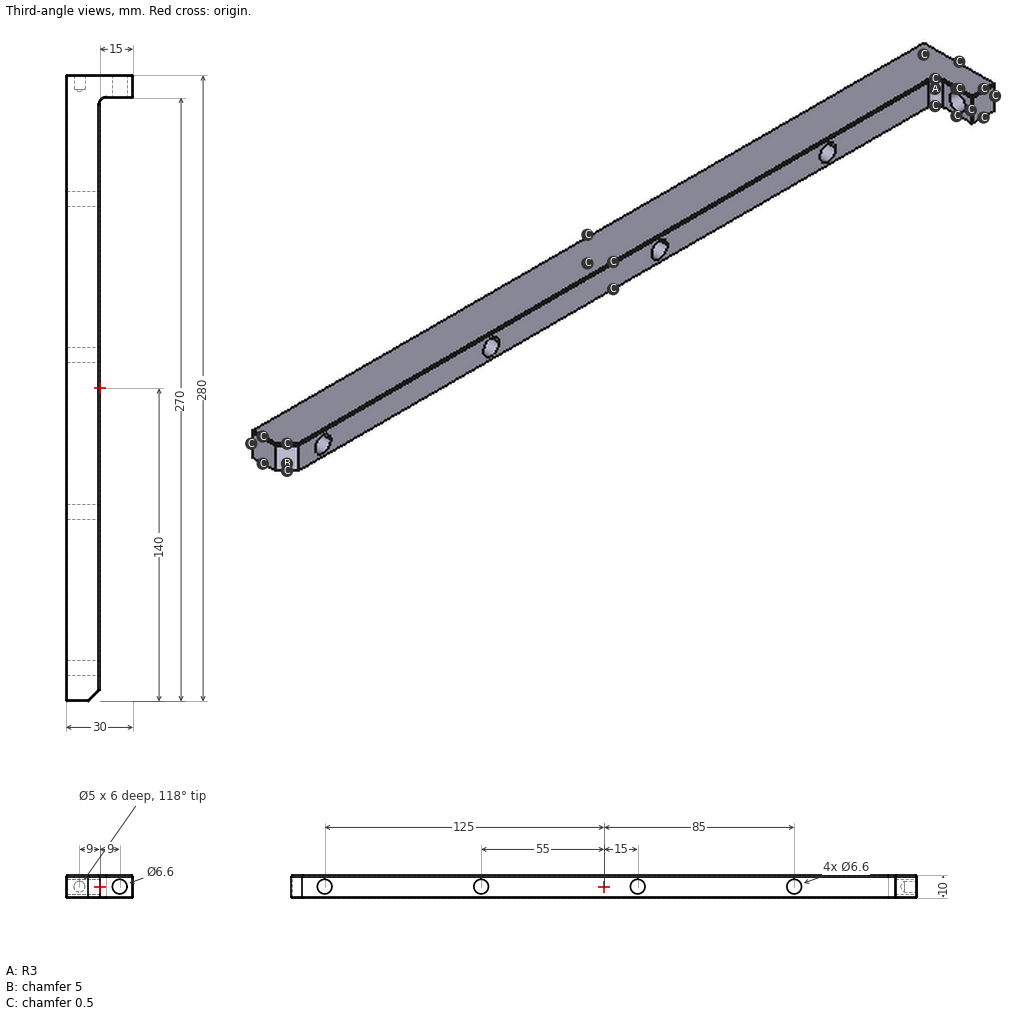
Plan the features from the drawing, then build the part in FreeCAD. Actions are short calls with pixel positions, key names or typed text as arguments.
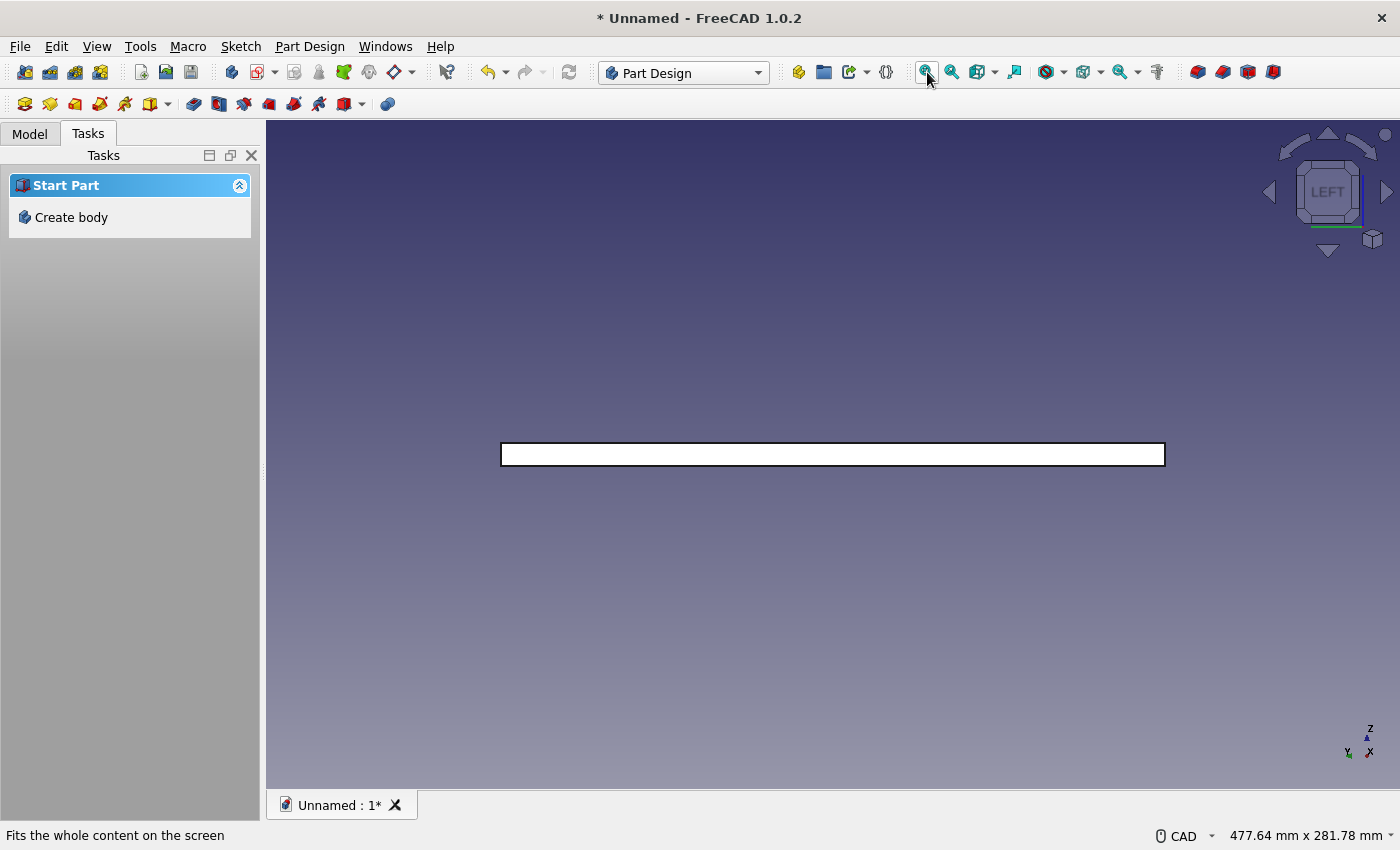
key(v)
key(3)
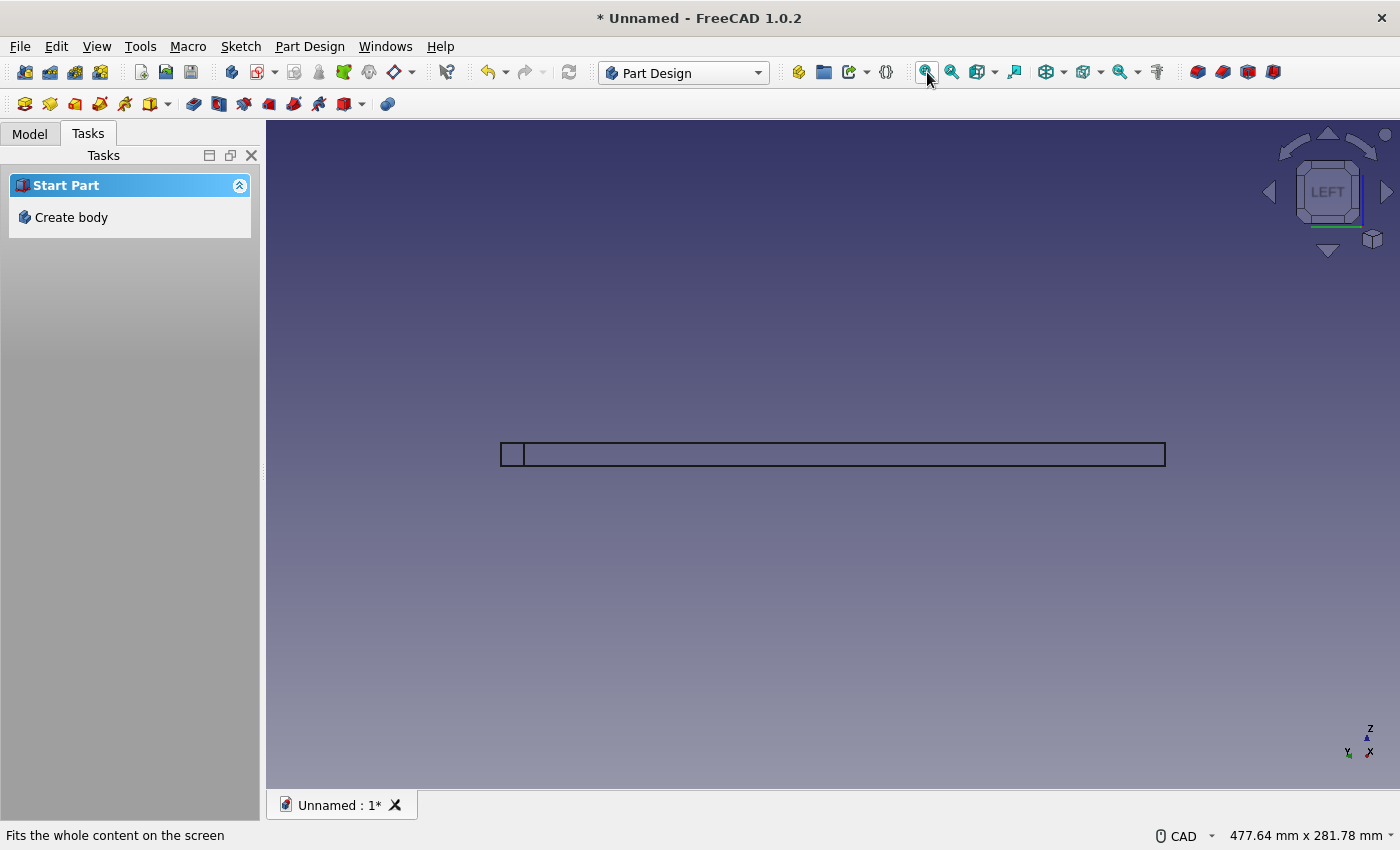
key(0)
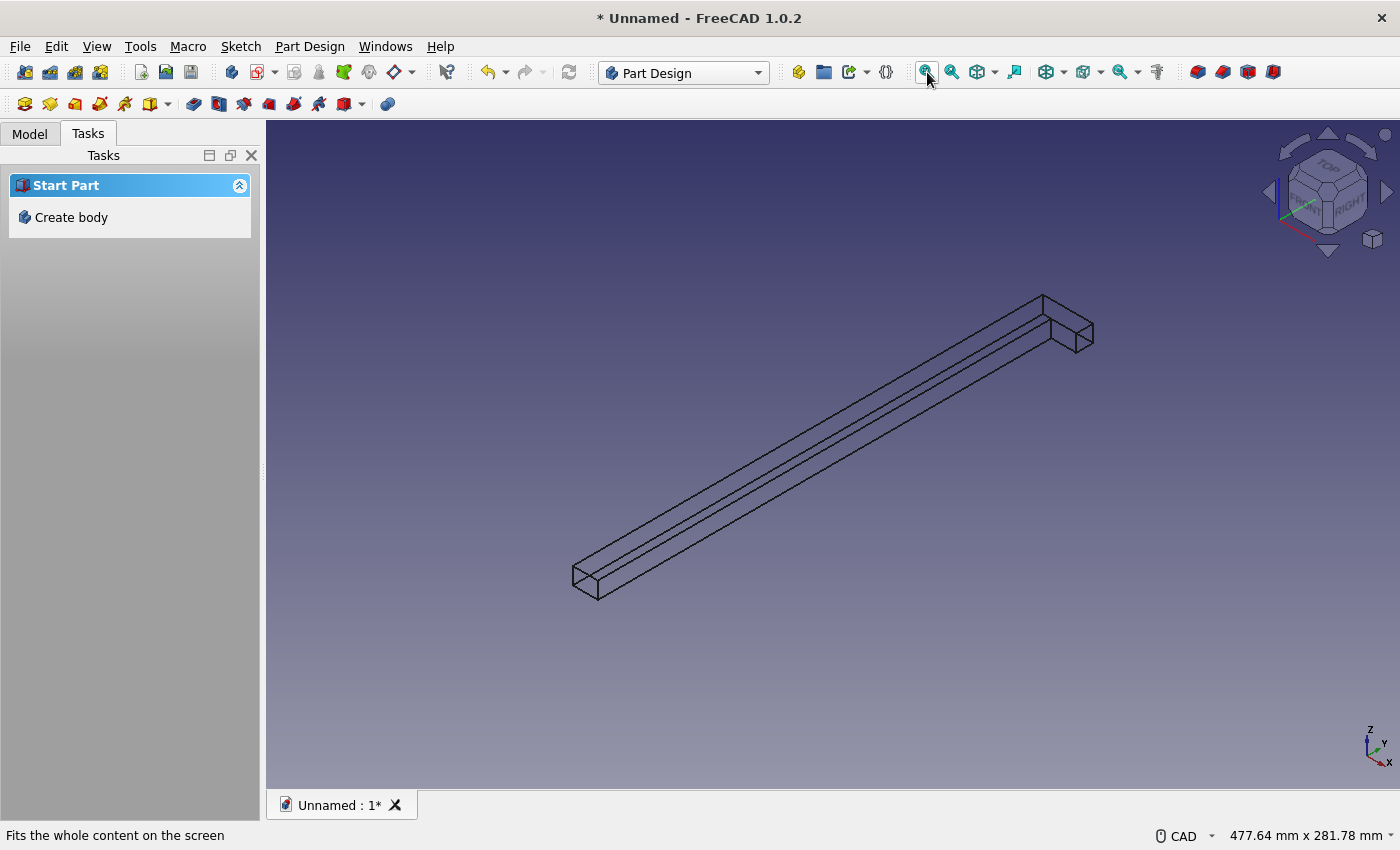
click(1051, 327)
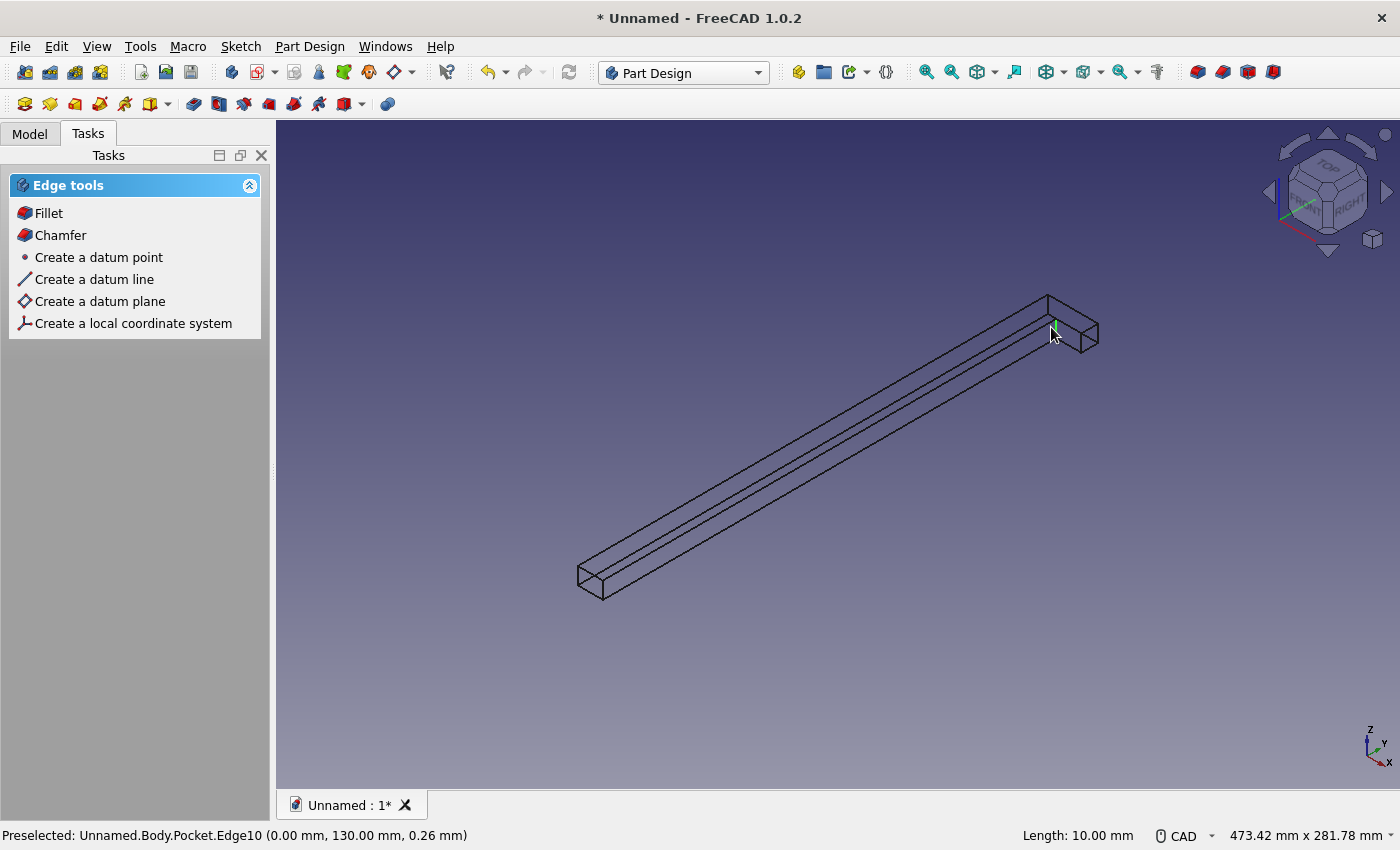
key(v)
key(1)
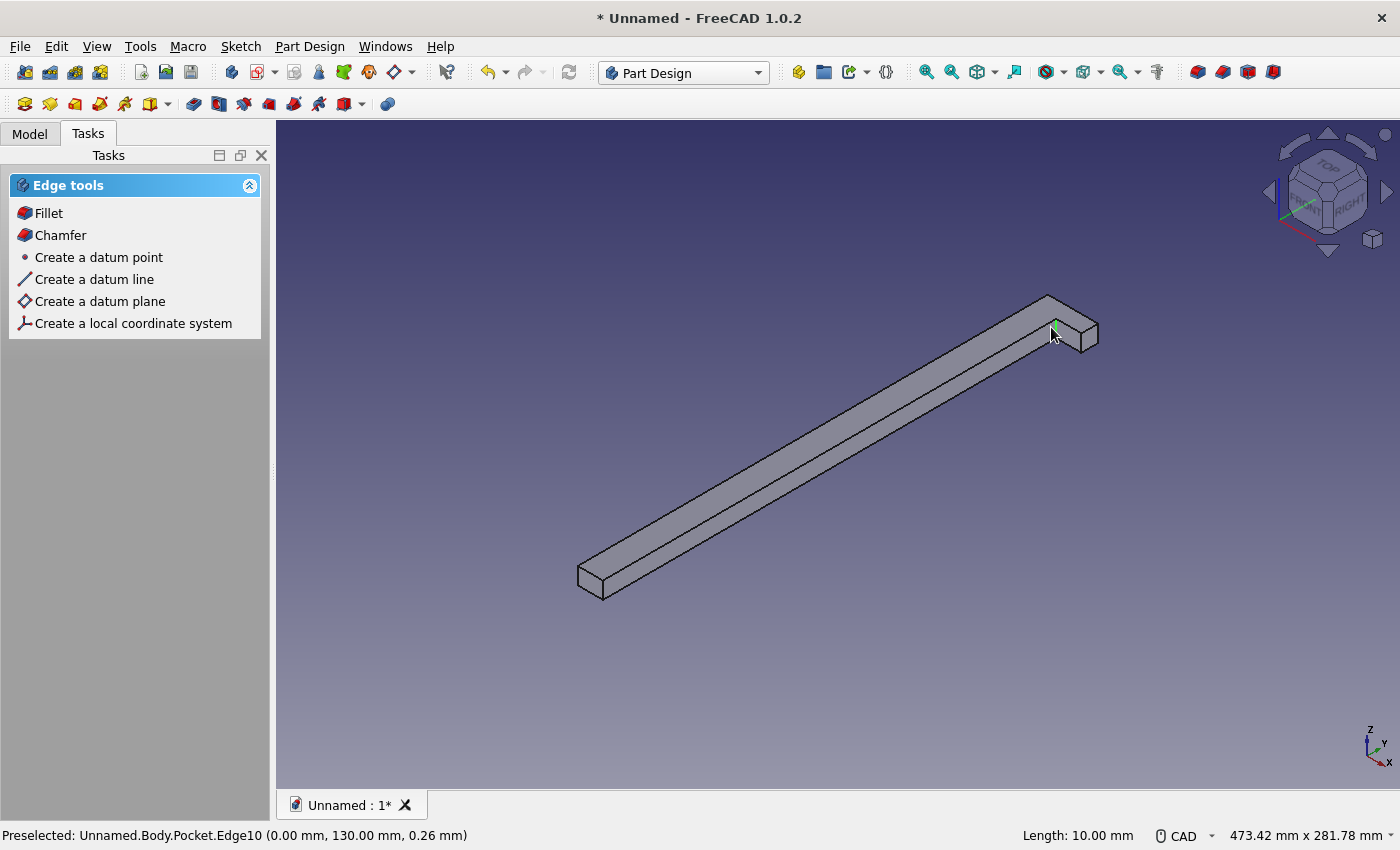
click(1198, 72)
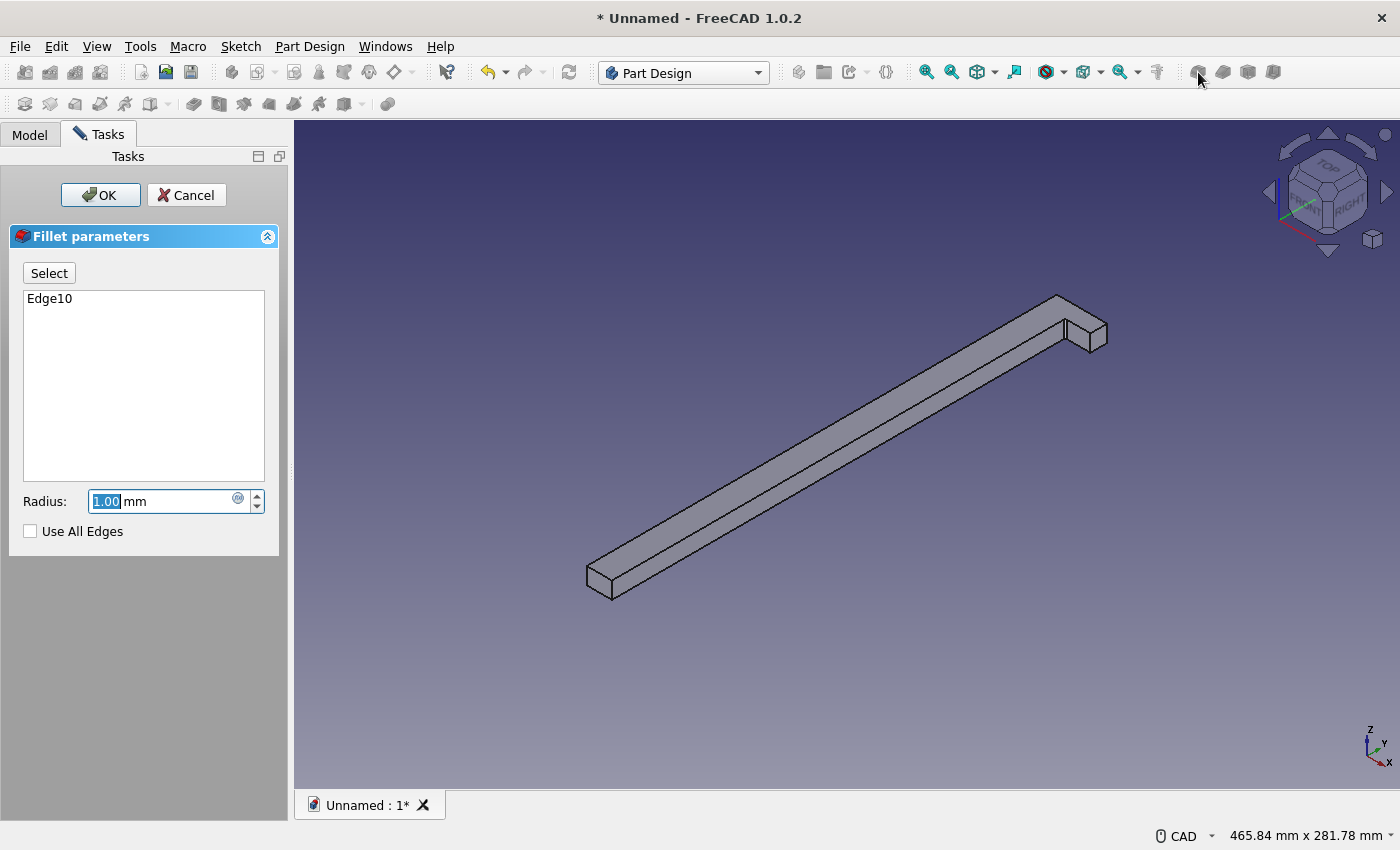
text(3)
key(Tab)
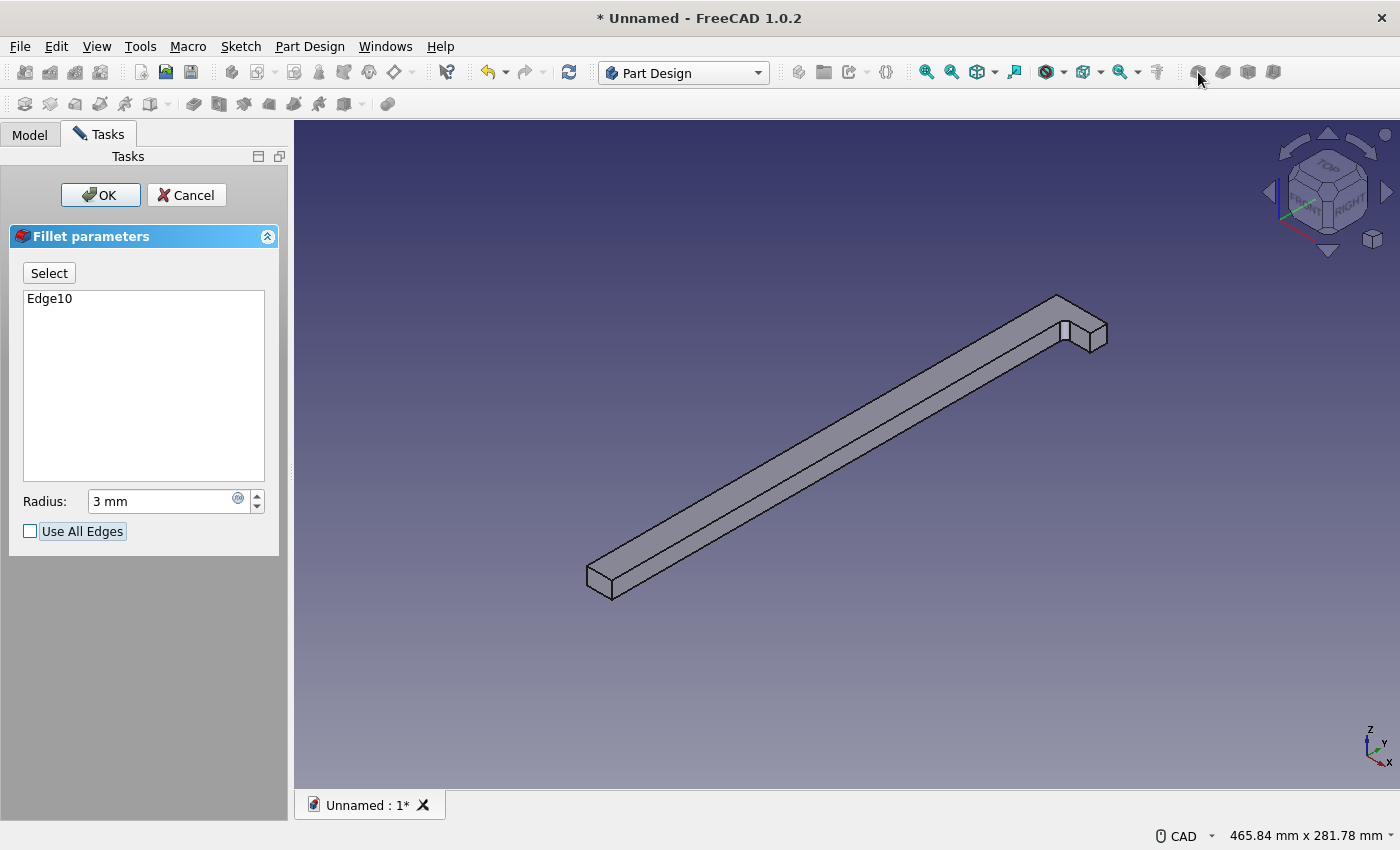
click(101, 195)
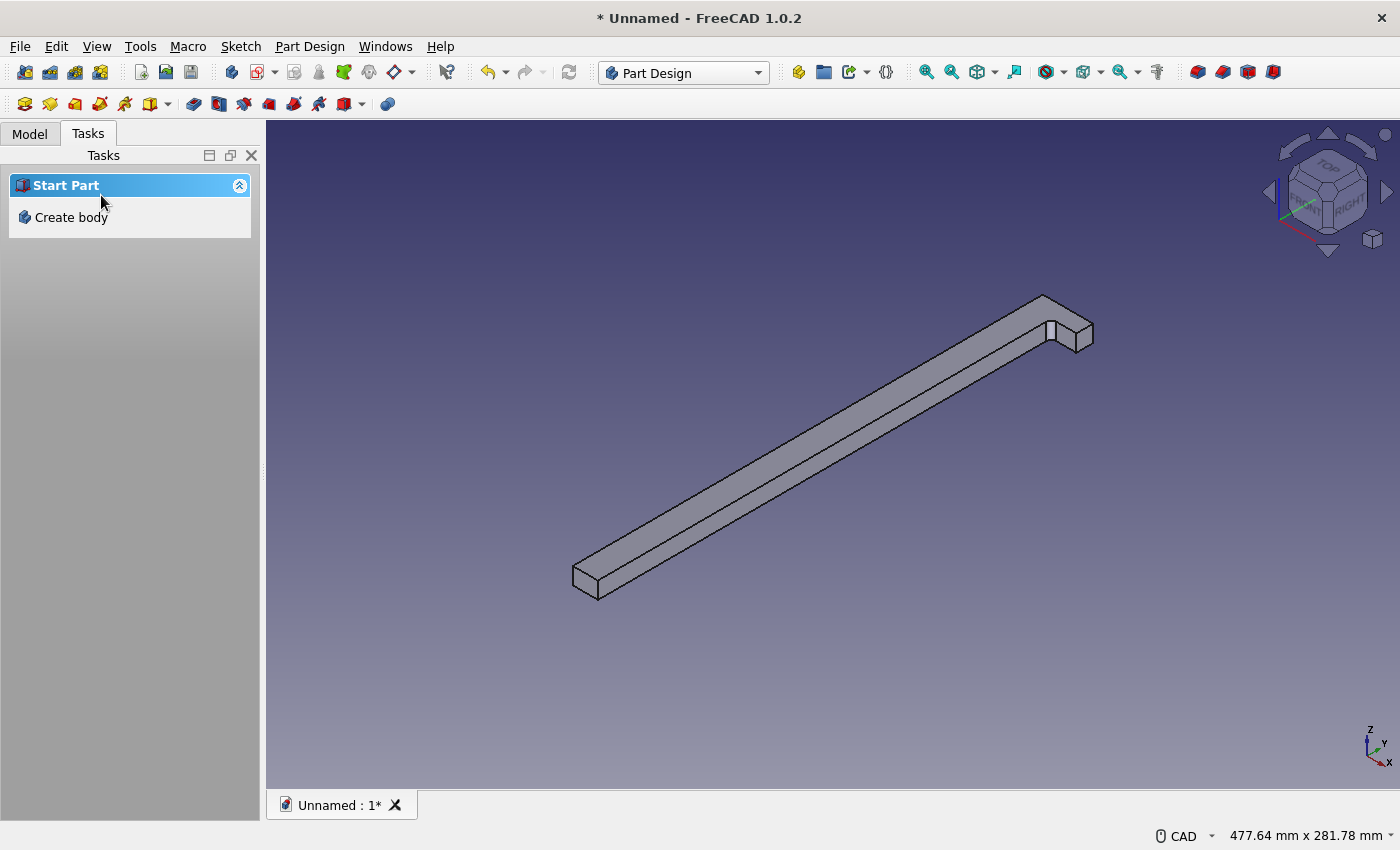
click(1066, 339)